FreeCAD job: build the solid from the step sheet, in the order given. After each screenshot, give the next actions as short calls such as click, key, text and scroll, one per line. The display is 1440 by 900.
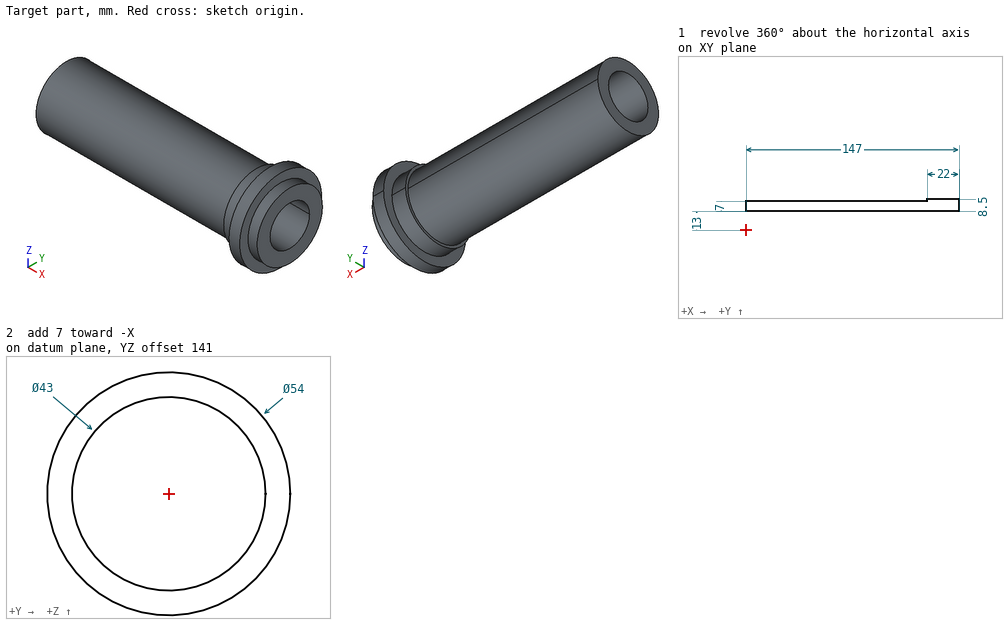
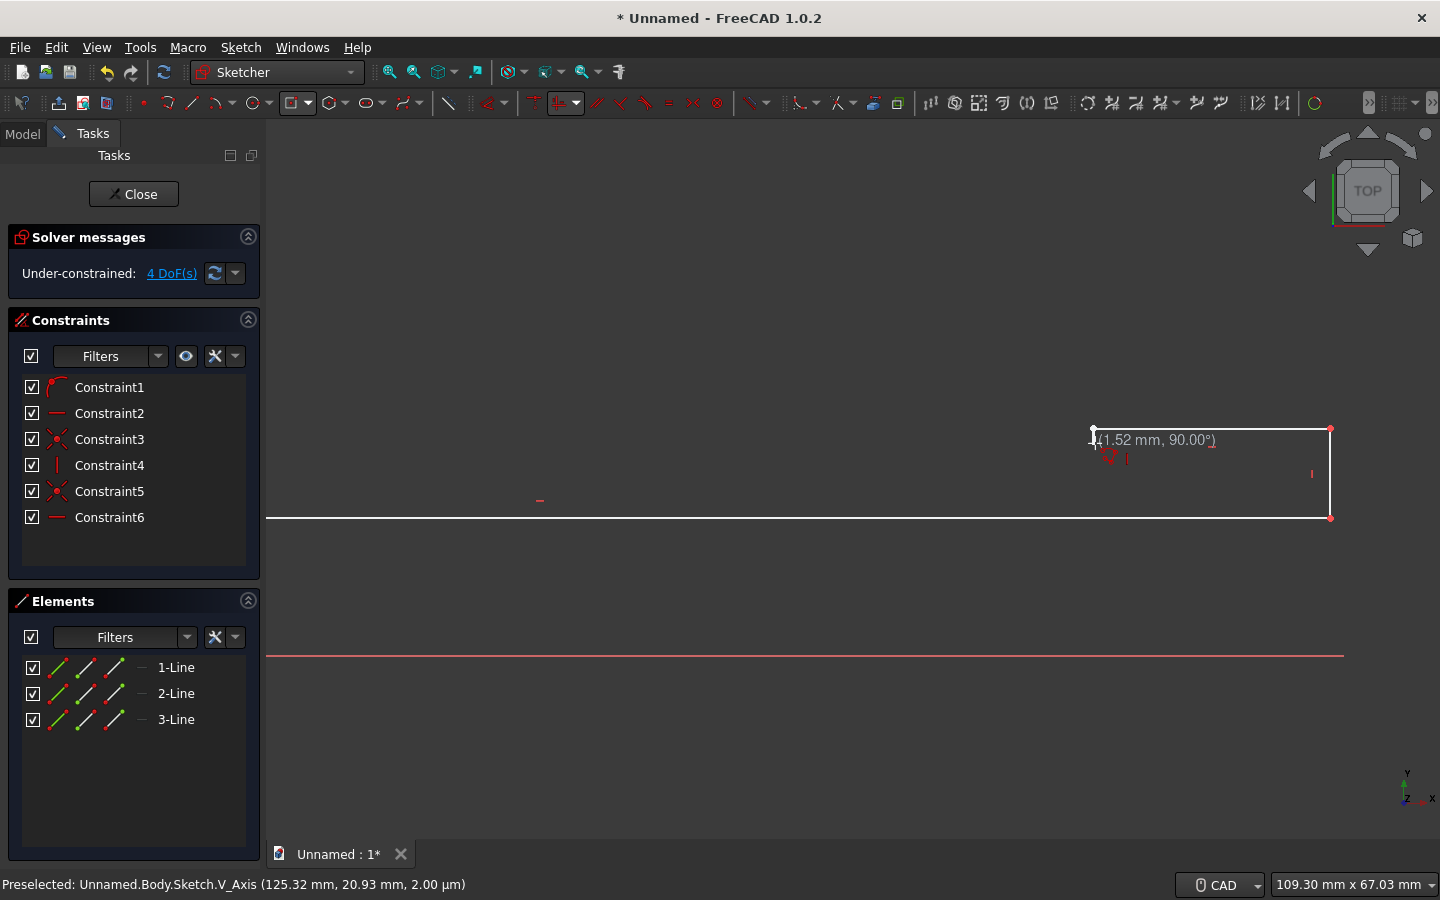
click(1094, 441)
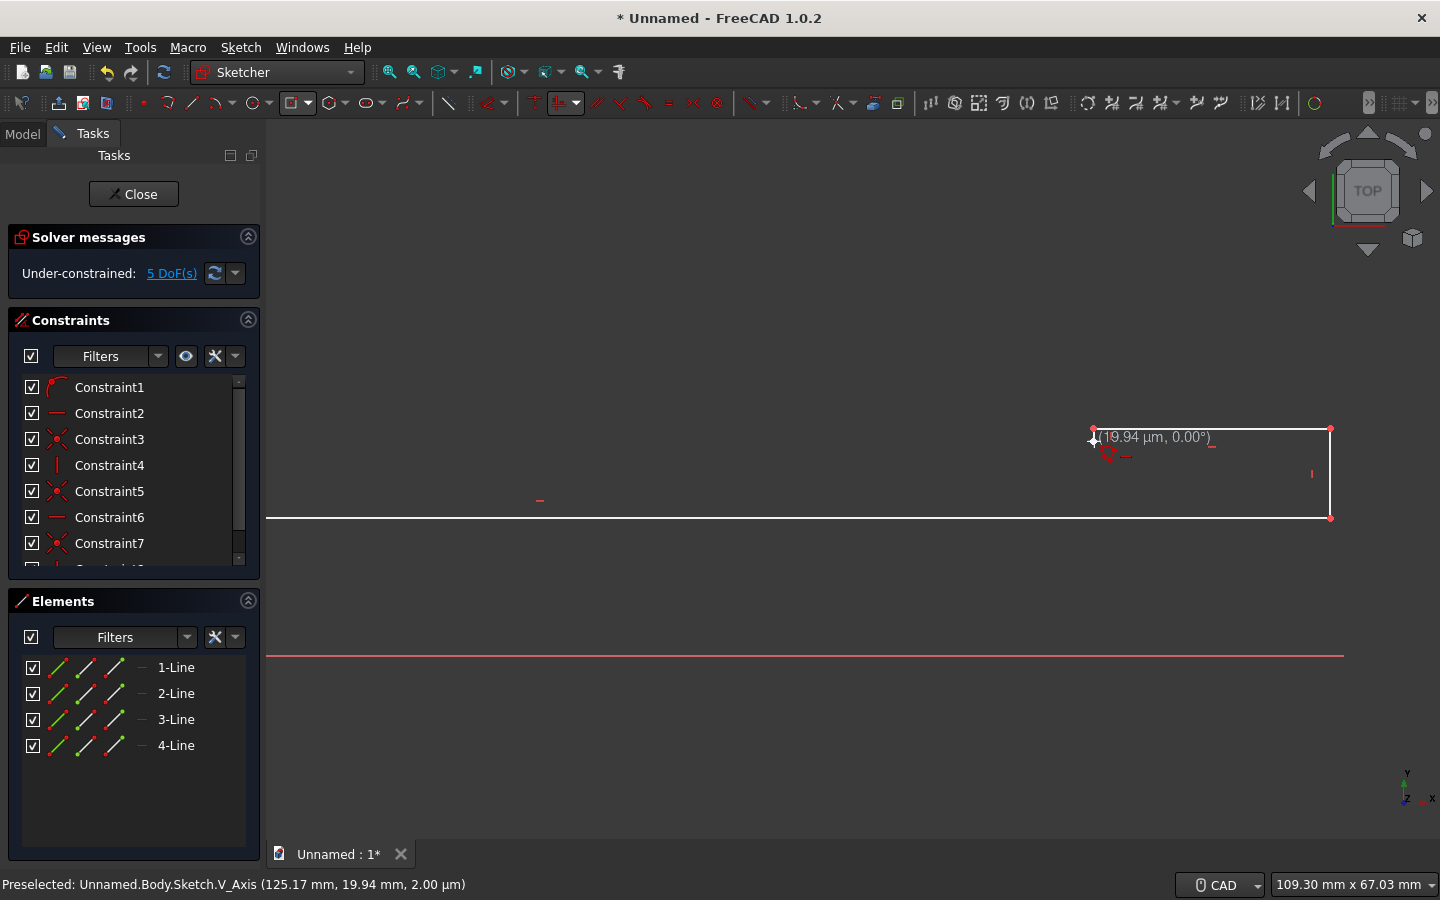
scroll(984, 429, down, 4)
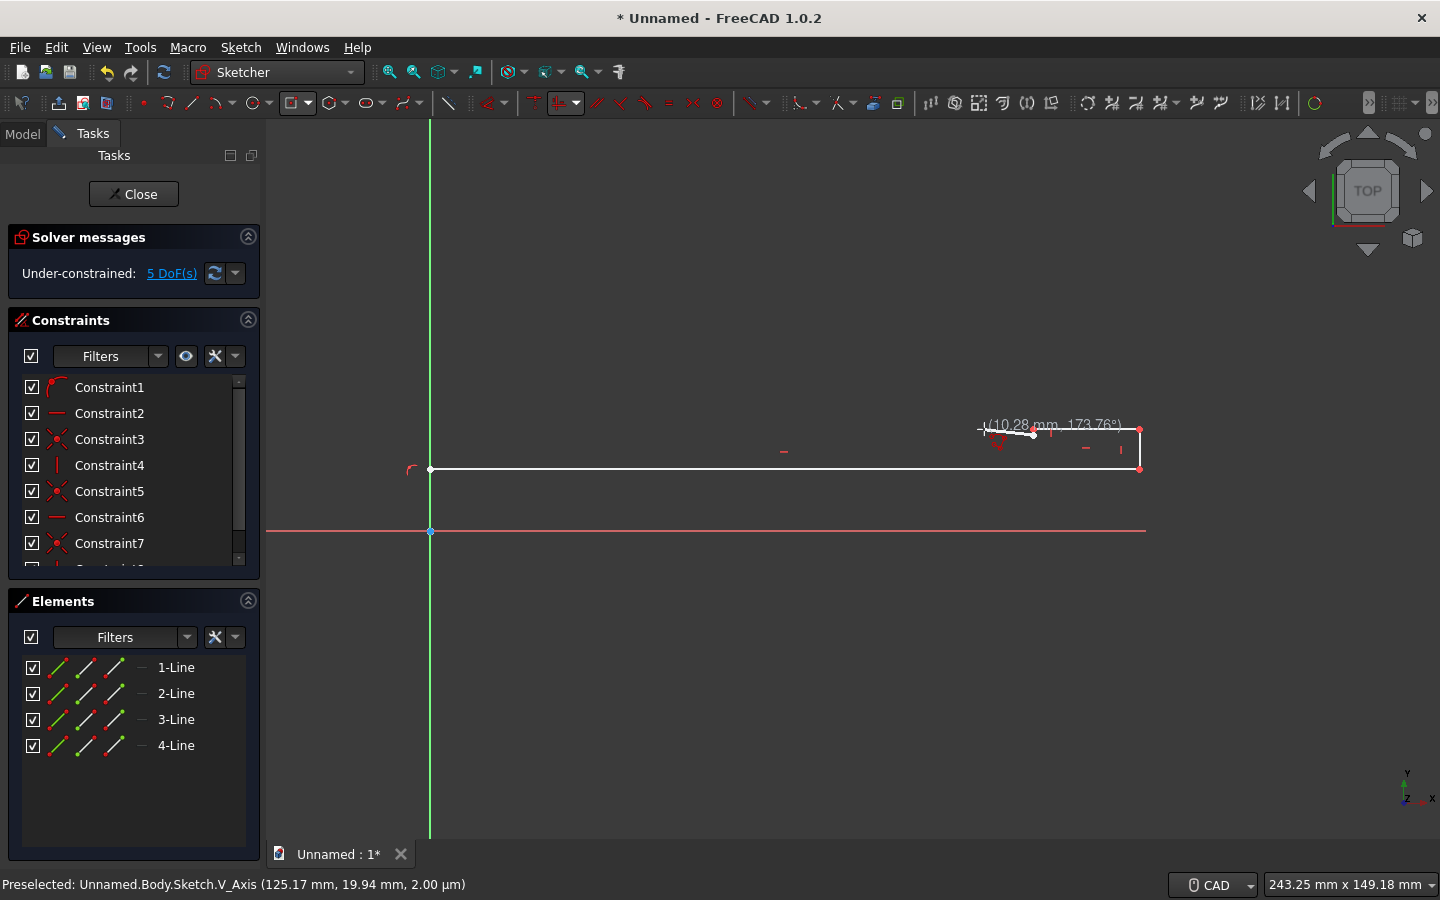
click(439, 435)
click(430, 469)
key(Escape)
key(Escape)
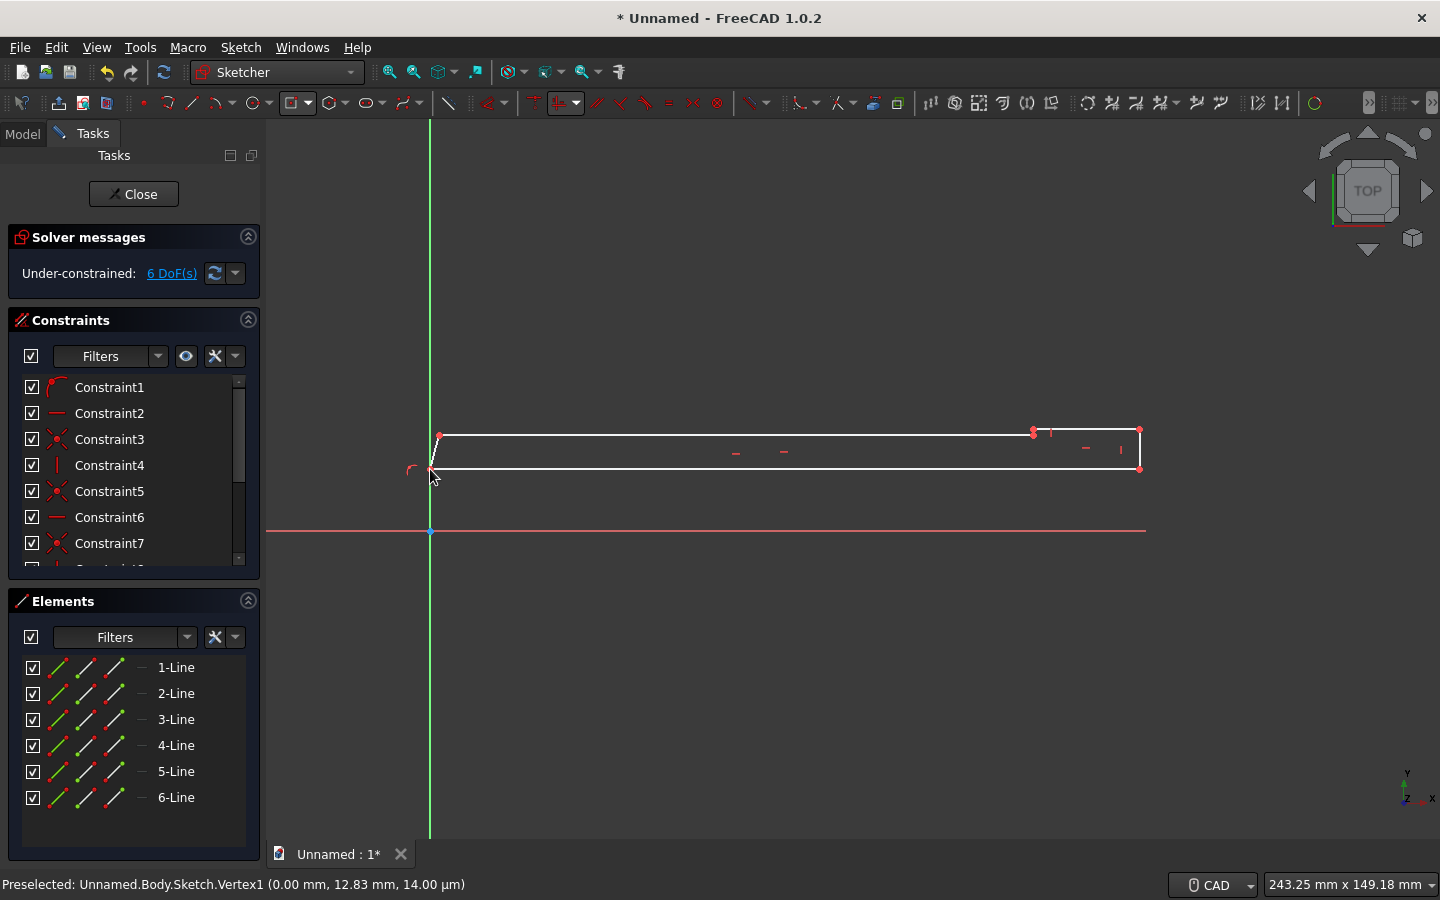
scroll(433, 459, up, 2)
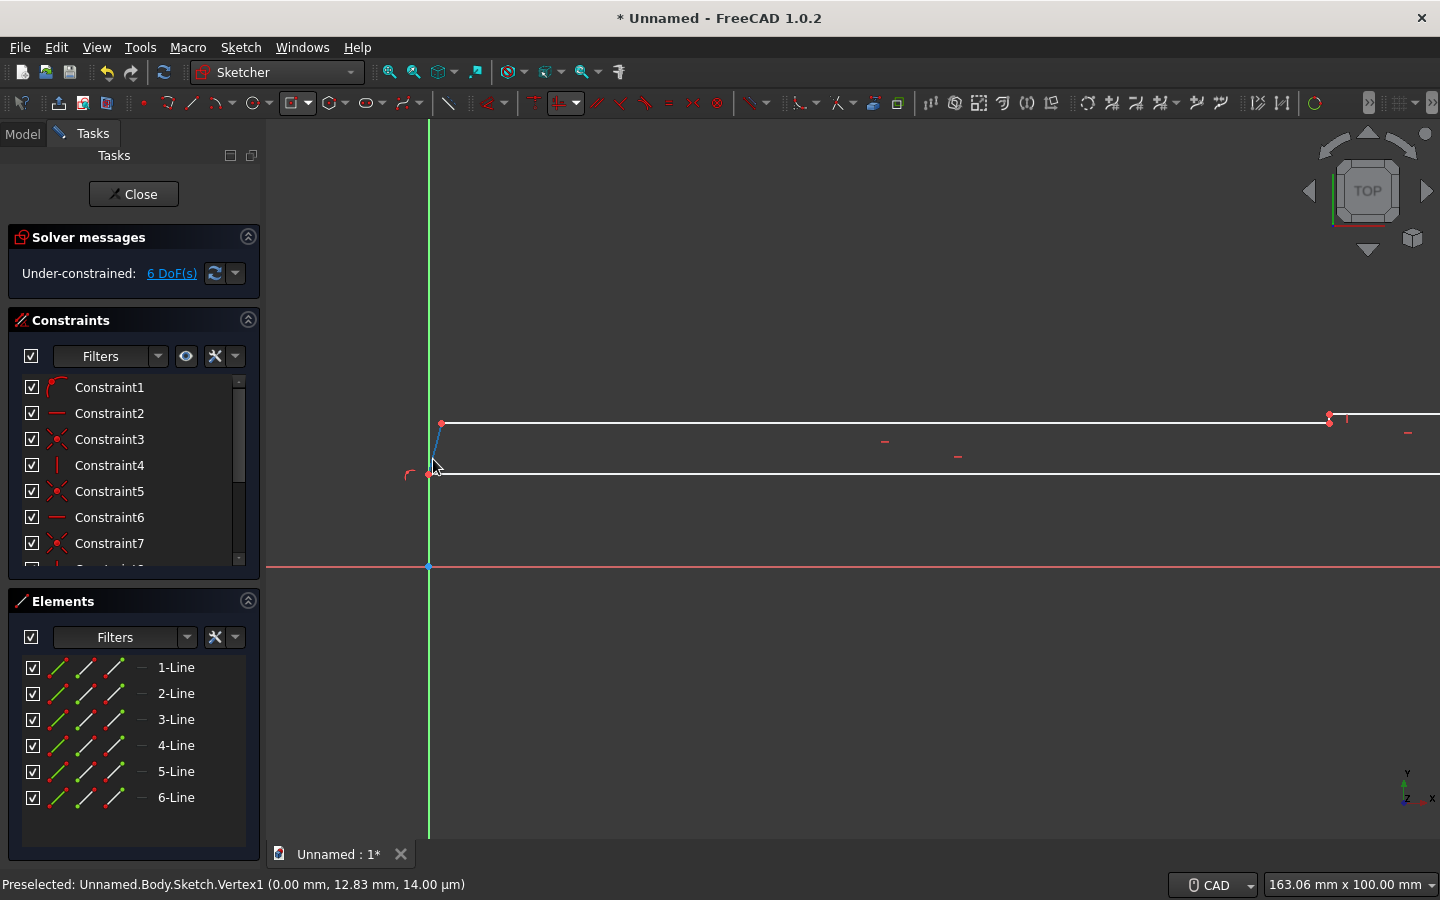
click(433, 459)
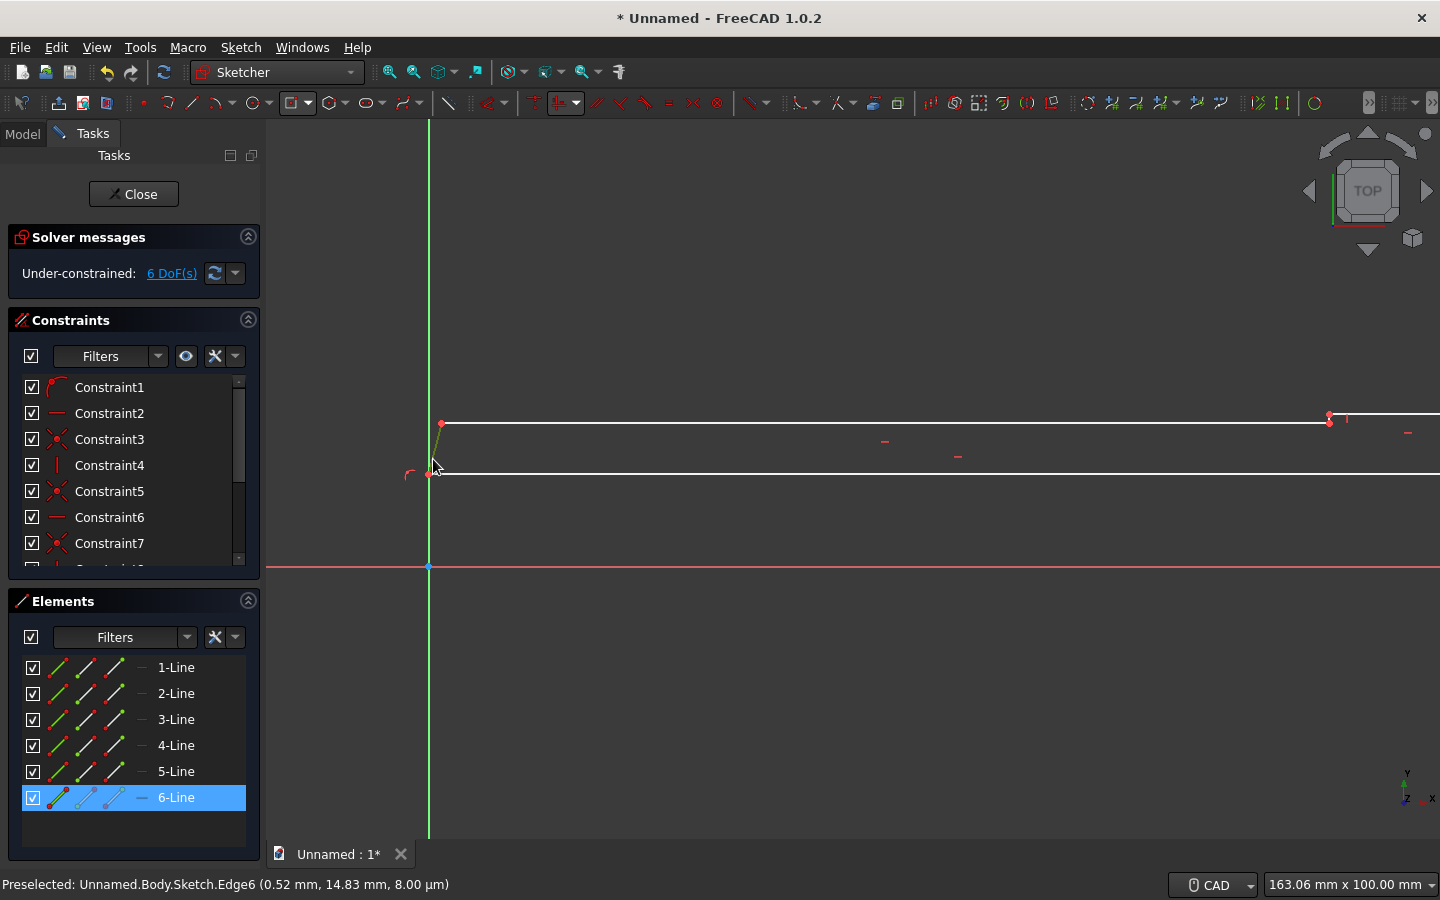
click(578, 104)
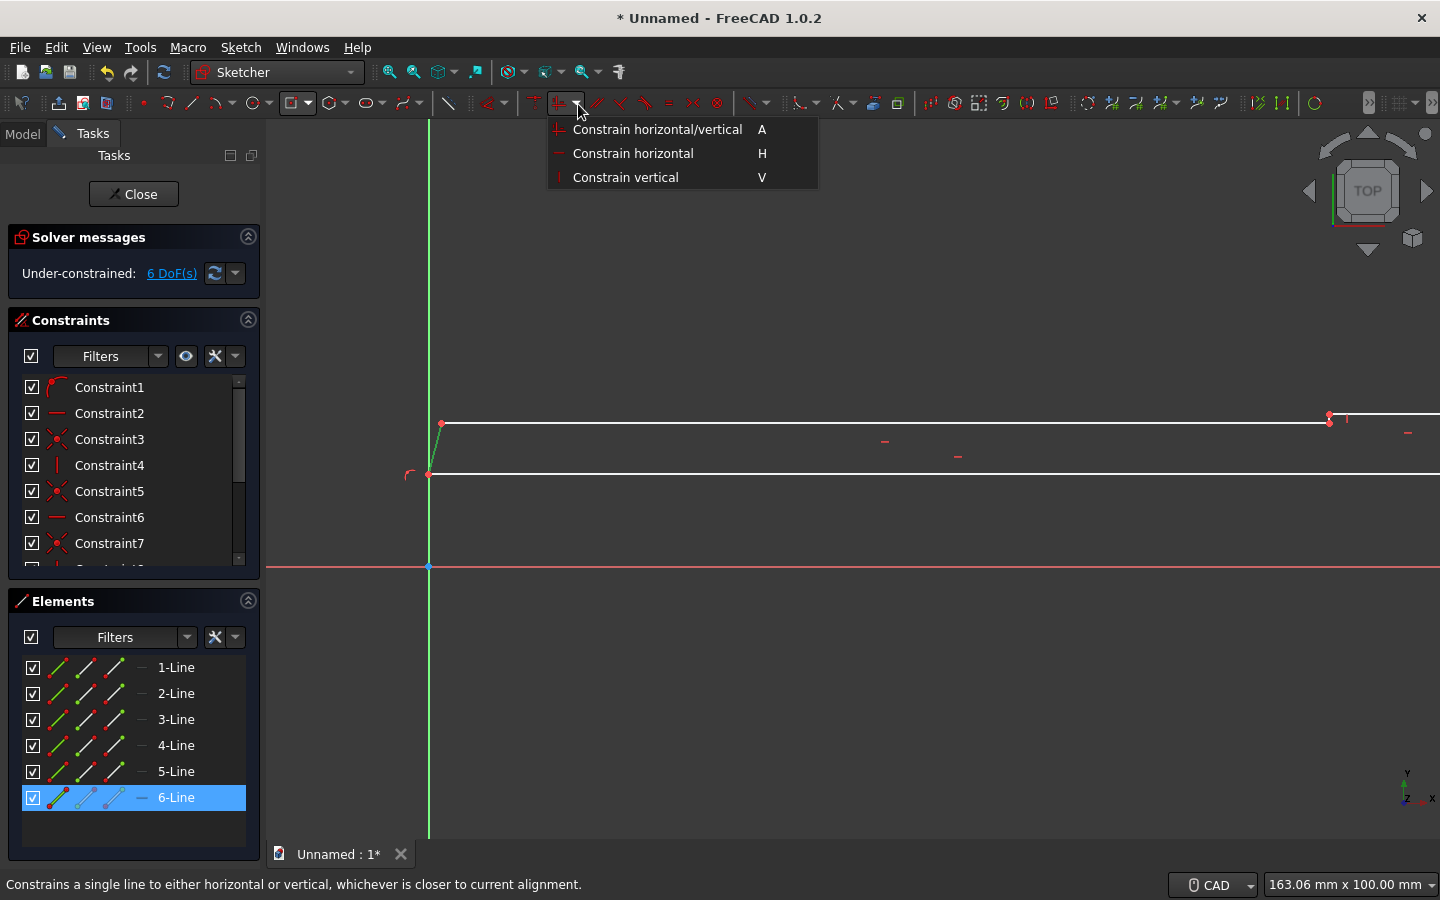
click(683, 177)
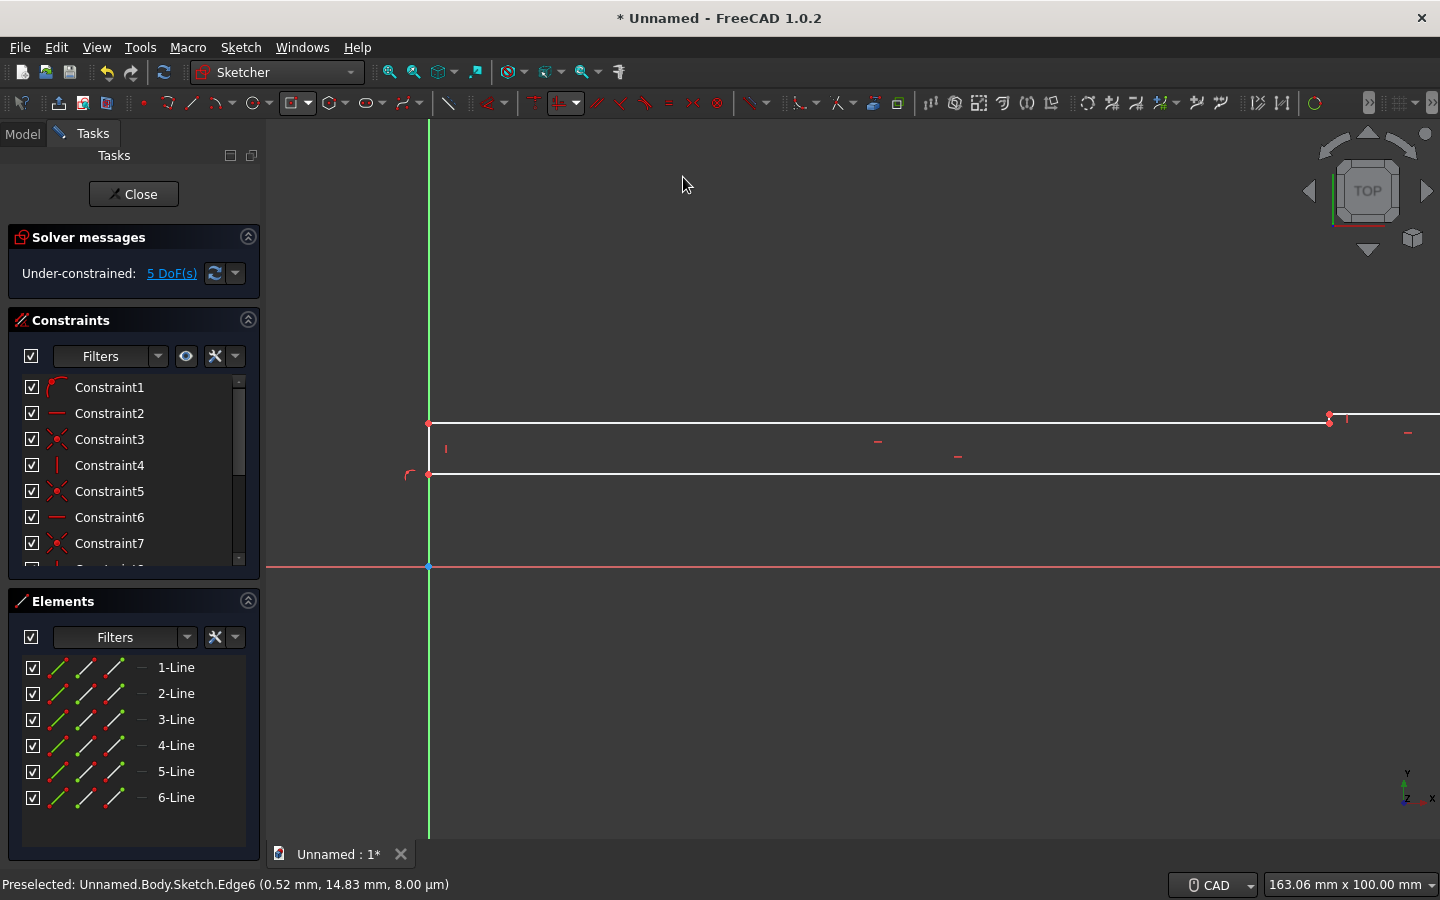
click(488, 104)